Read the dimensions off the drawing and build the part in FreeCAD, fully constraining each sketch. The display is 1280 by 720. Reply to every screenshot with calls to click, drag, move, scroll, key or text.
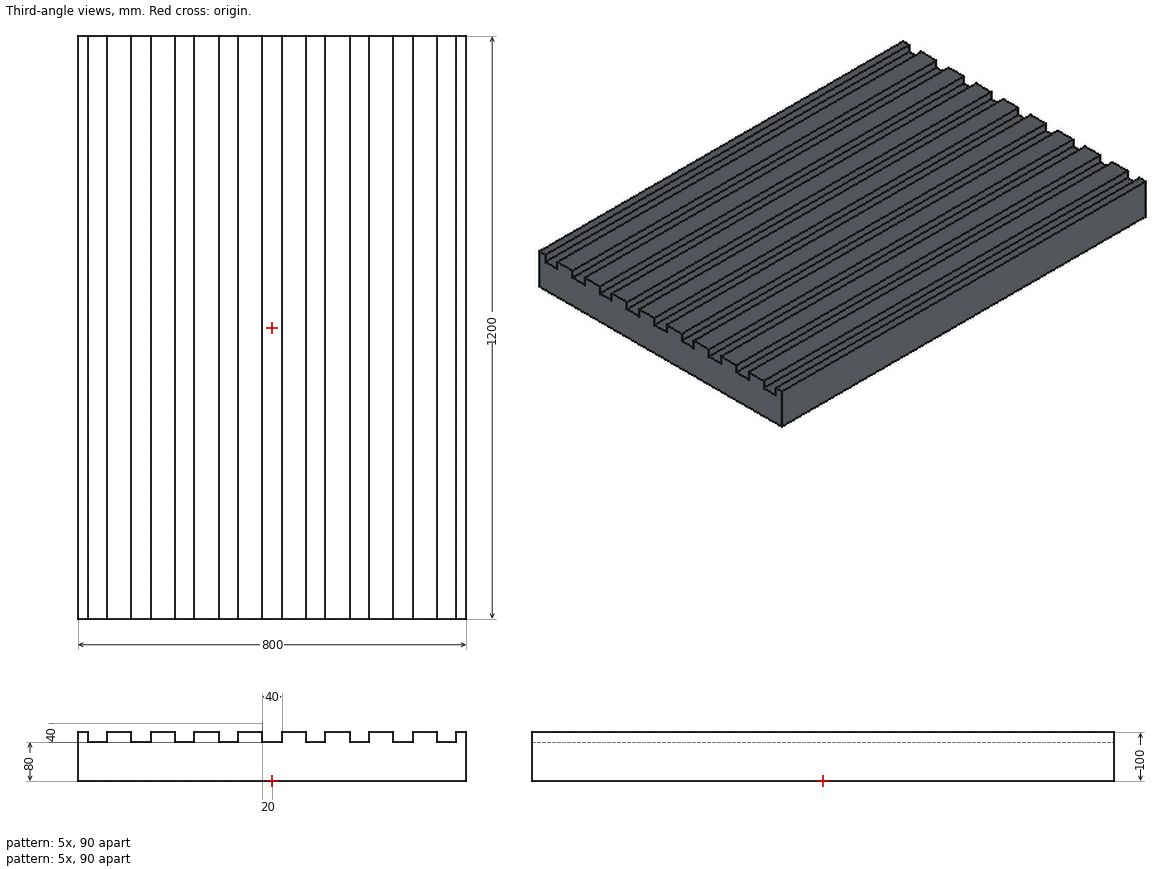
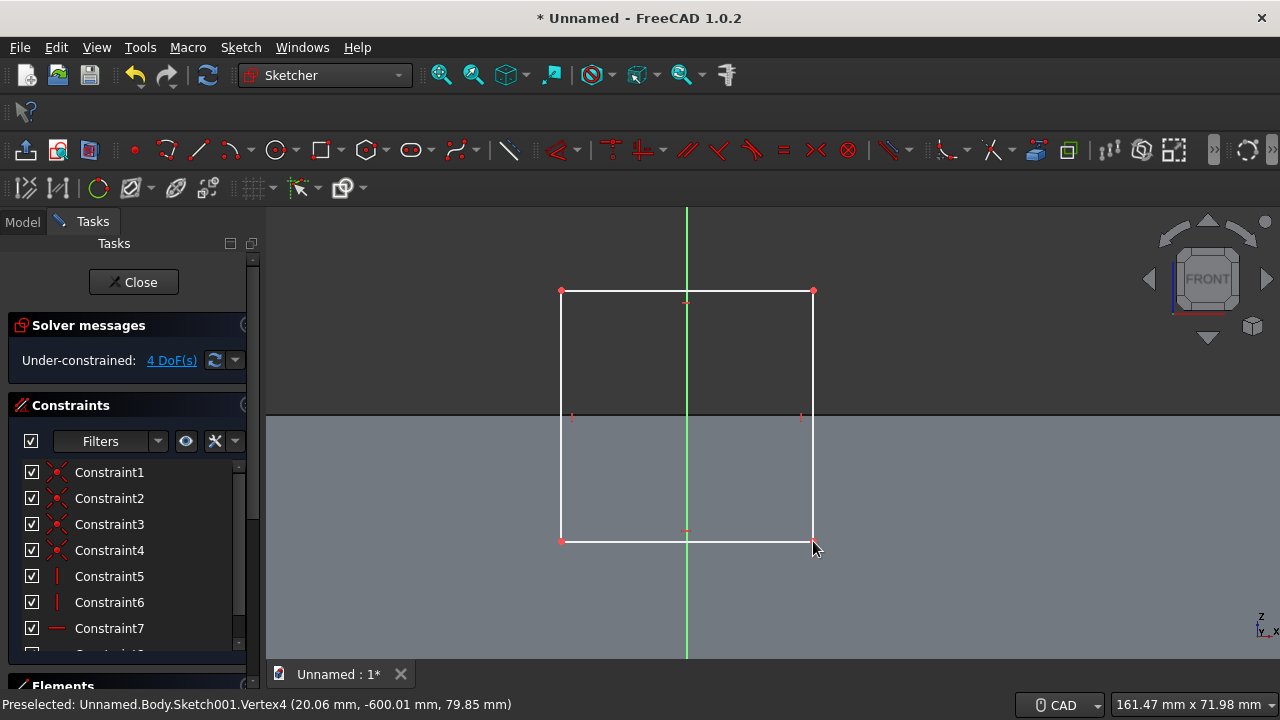
key(d)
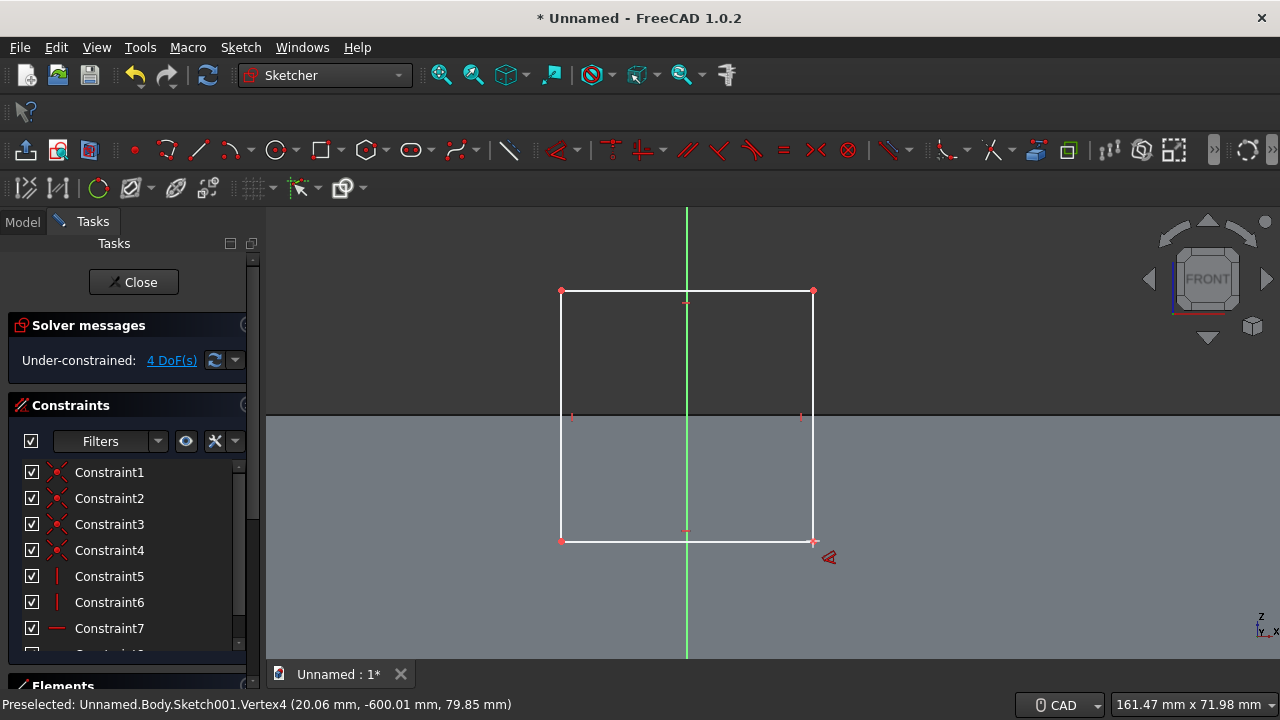
click(561, 366)
click(527, 416)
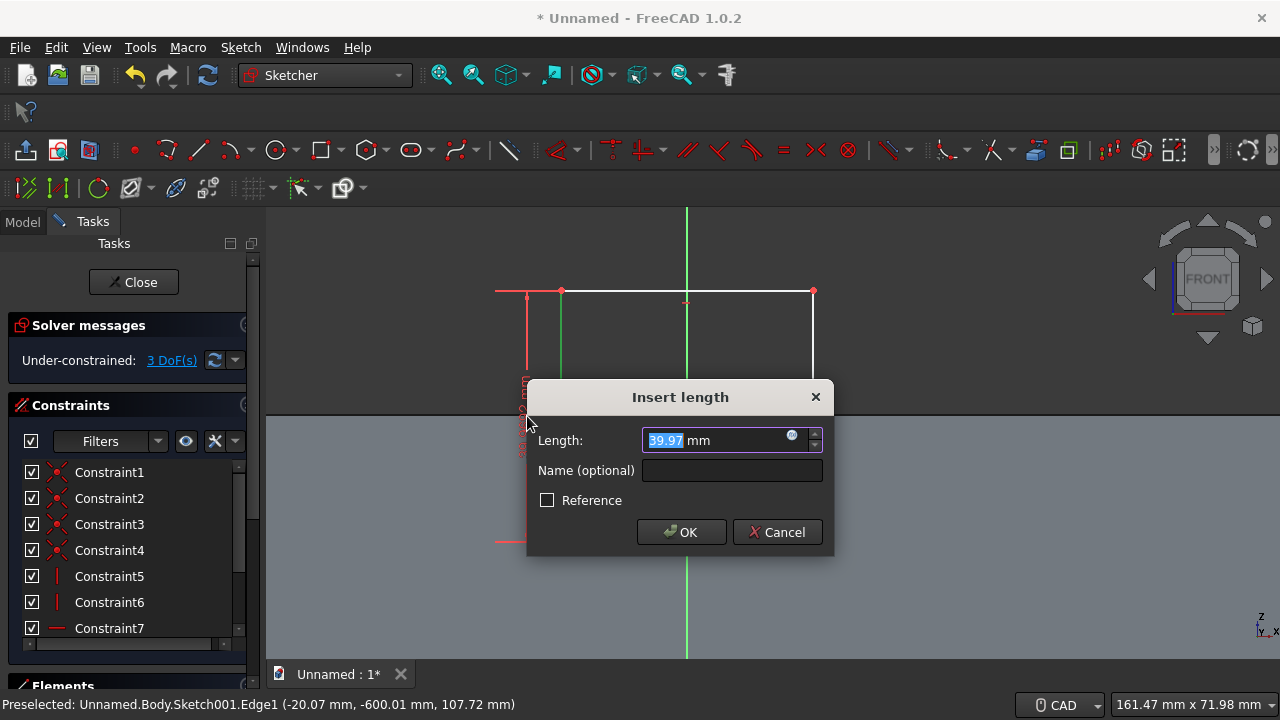
text(40)
key(Return)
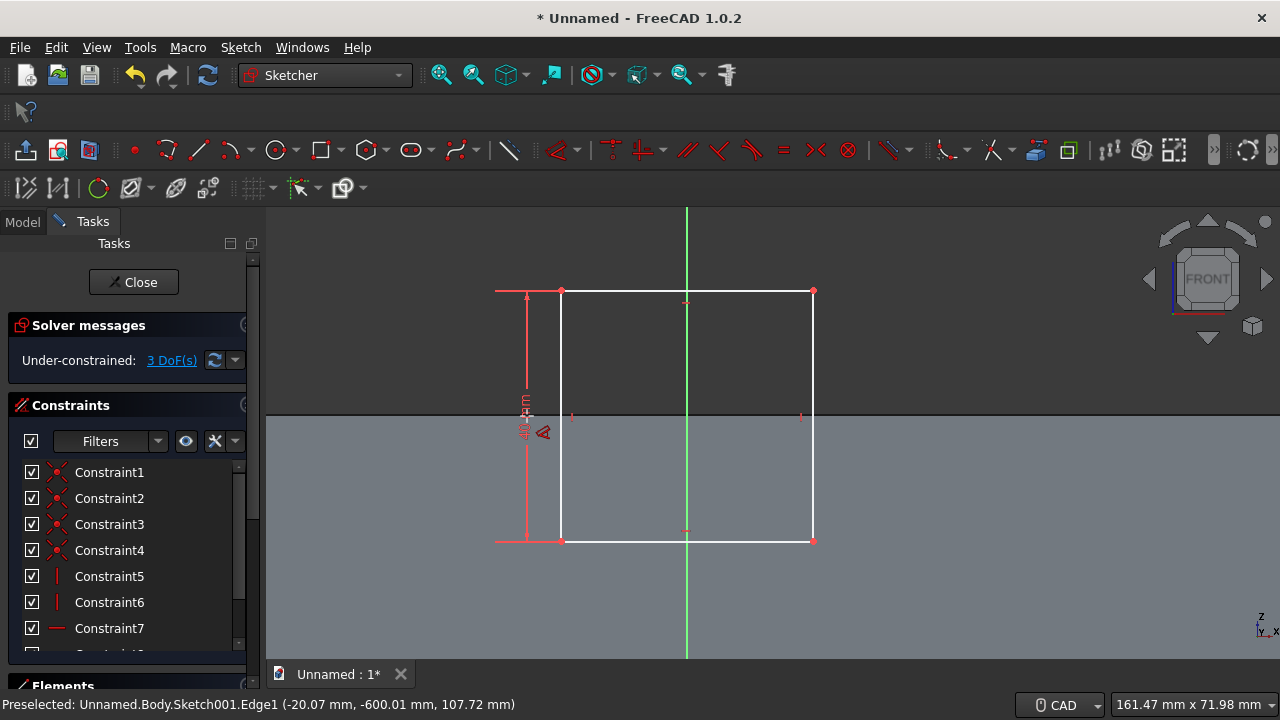
click(637, 542)
click(629, 576)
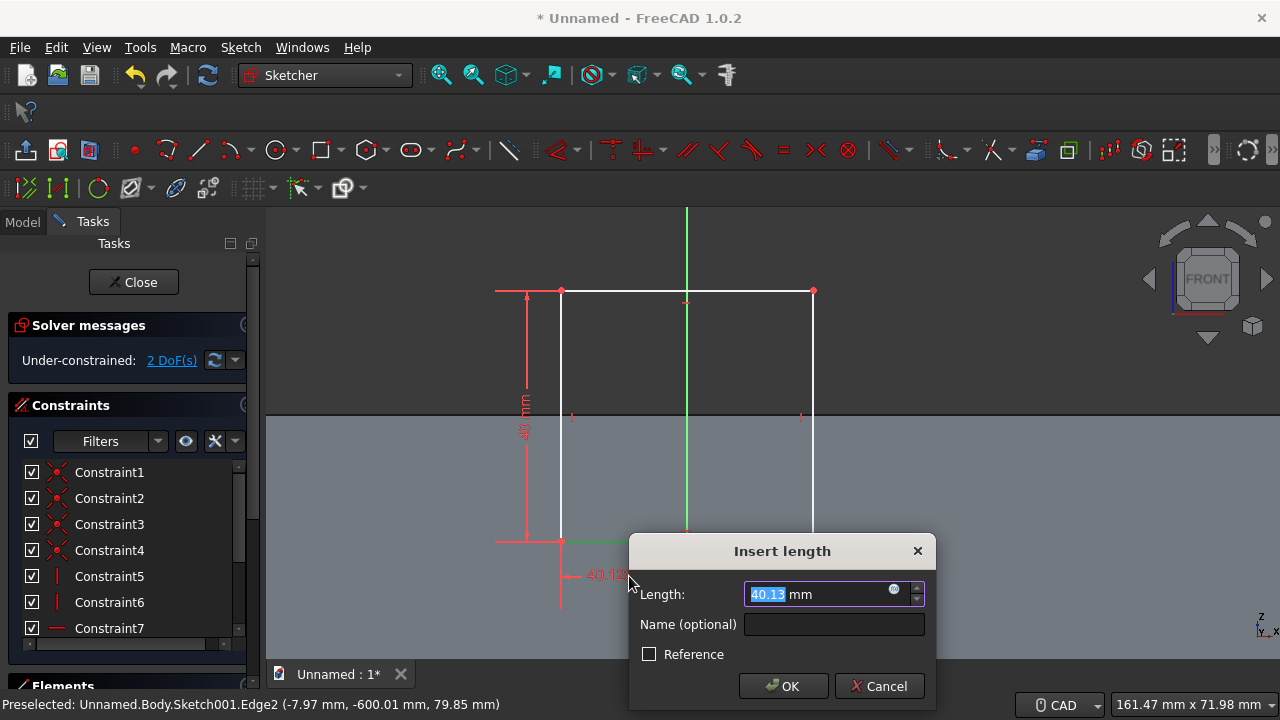
text(40)
key(Return)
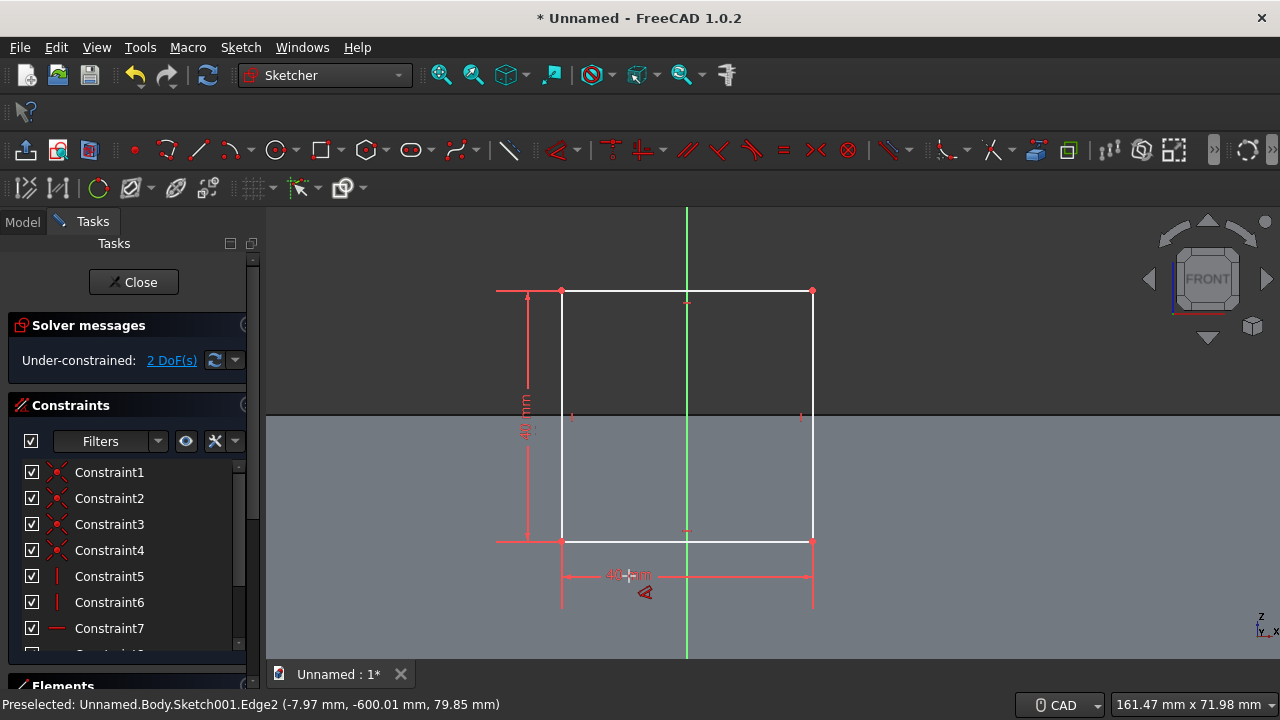
click(562, 291)
click(624, 257)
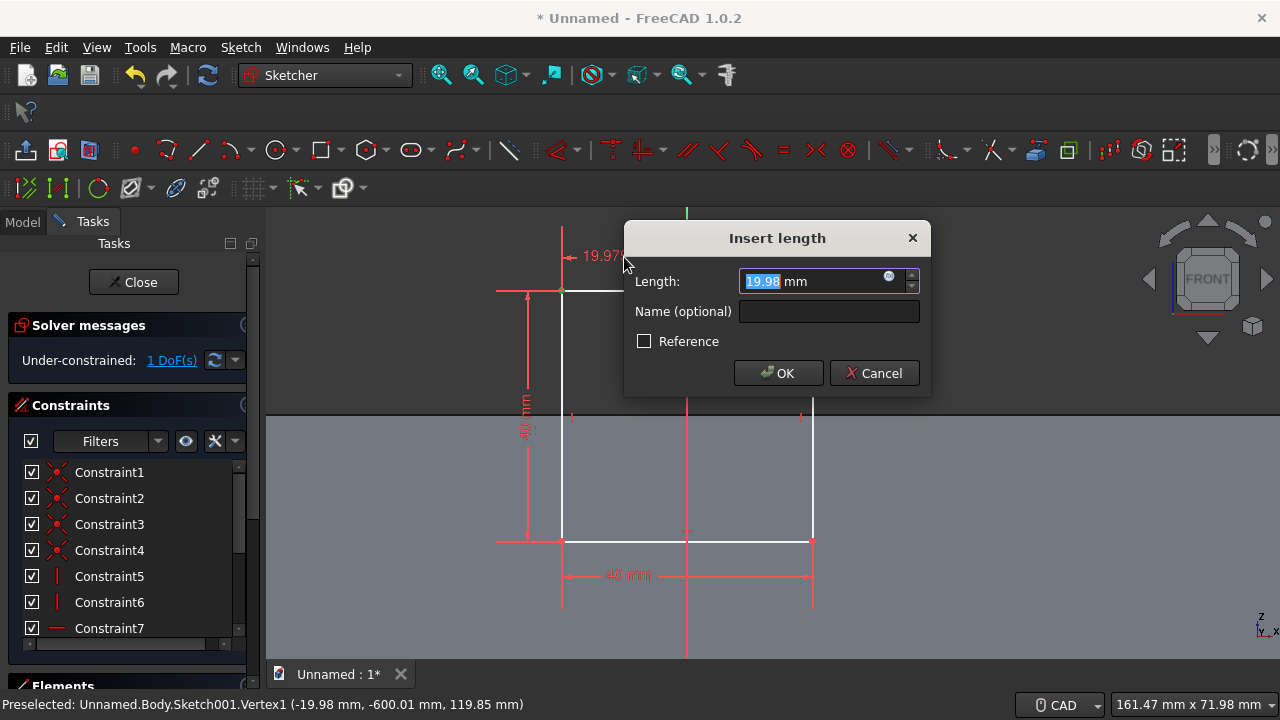
text(20)
key(Return)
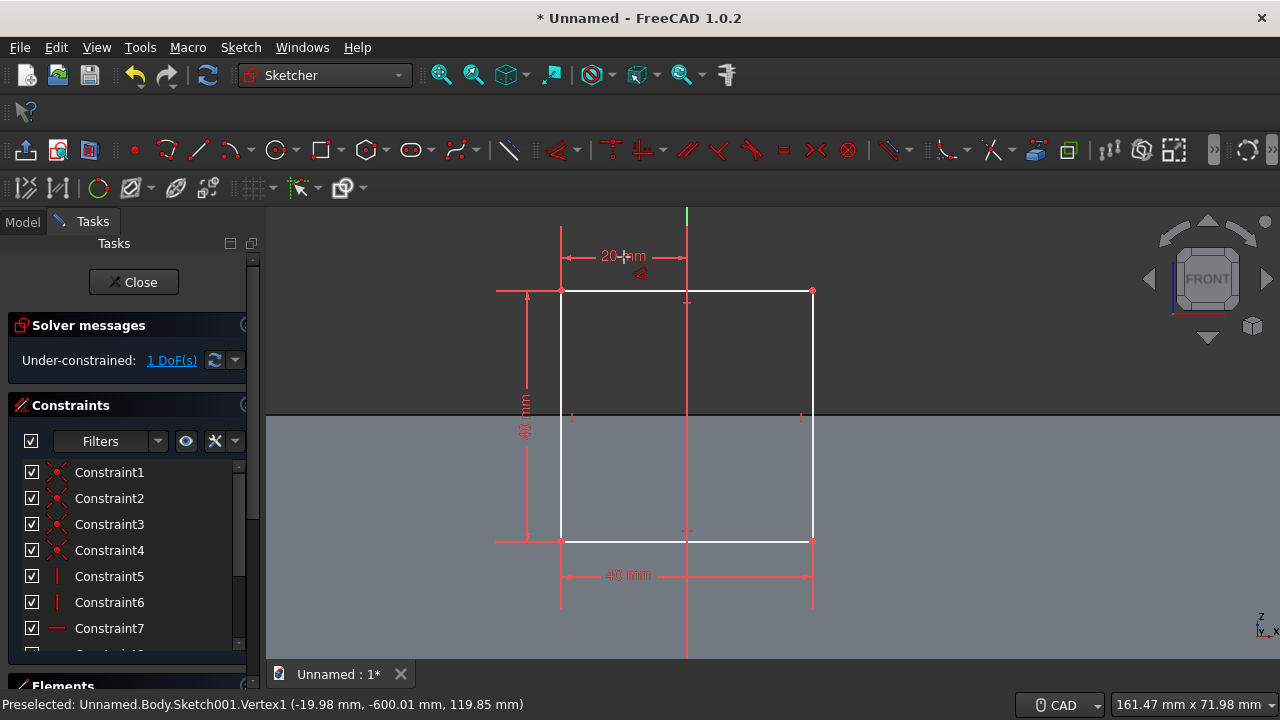
click(561, 542)
click(527, 586)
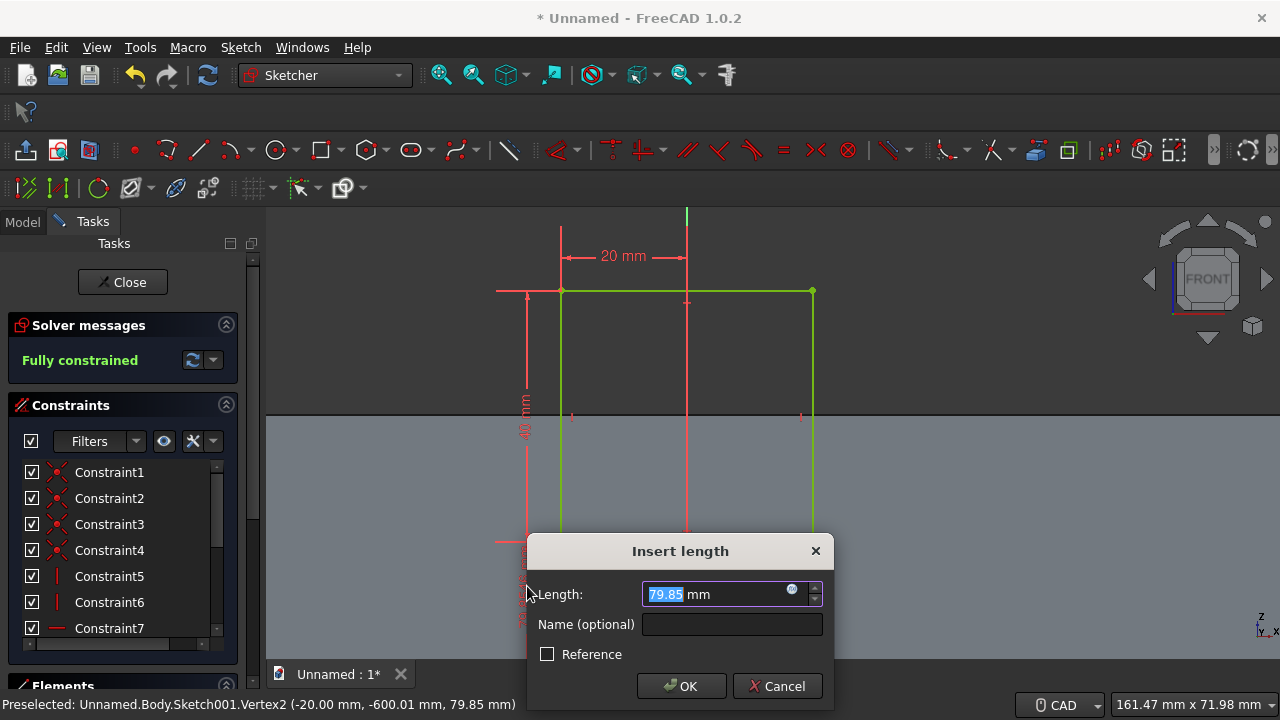
text(80)
key(Return)
key(Escape)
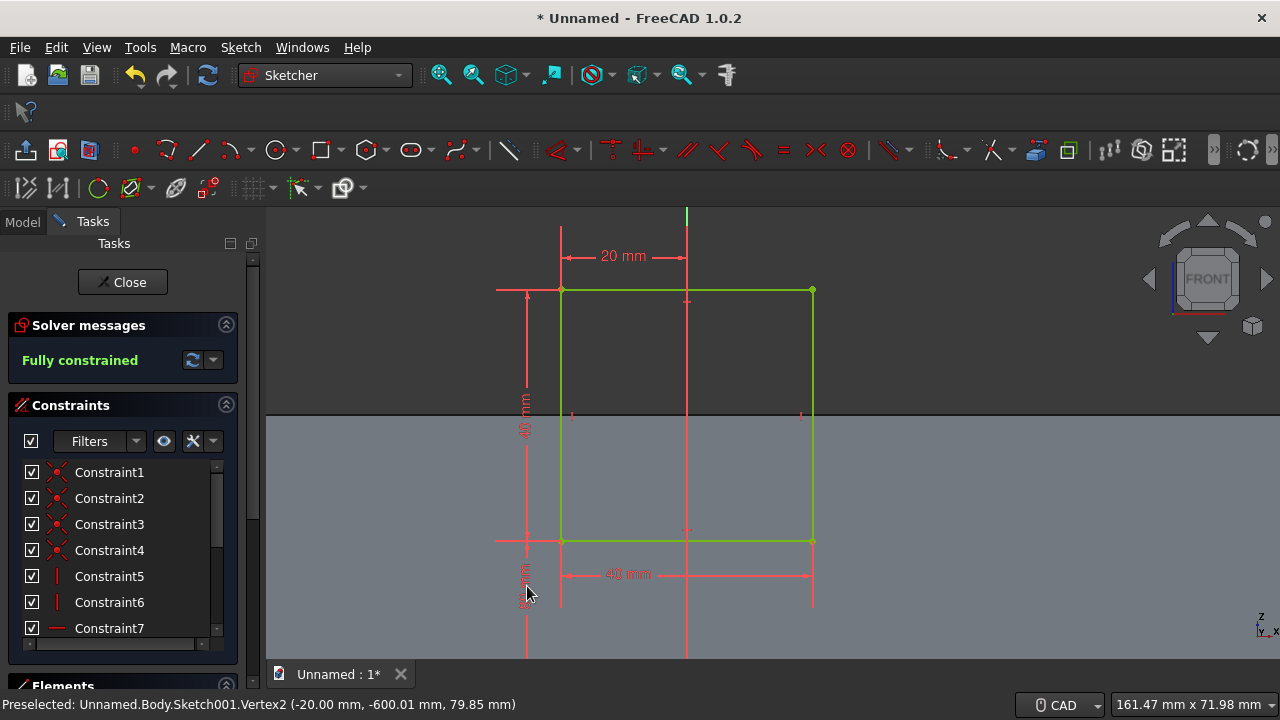
click(123, 282)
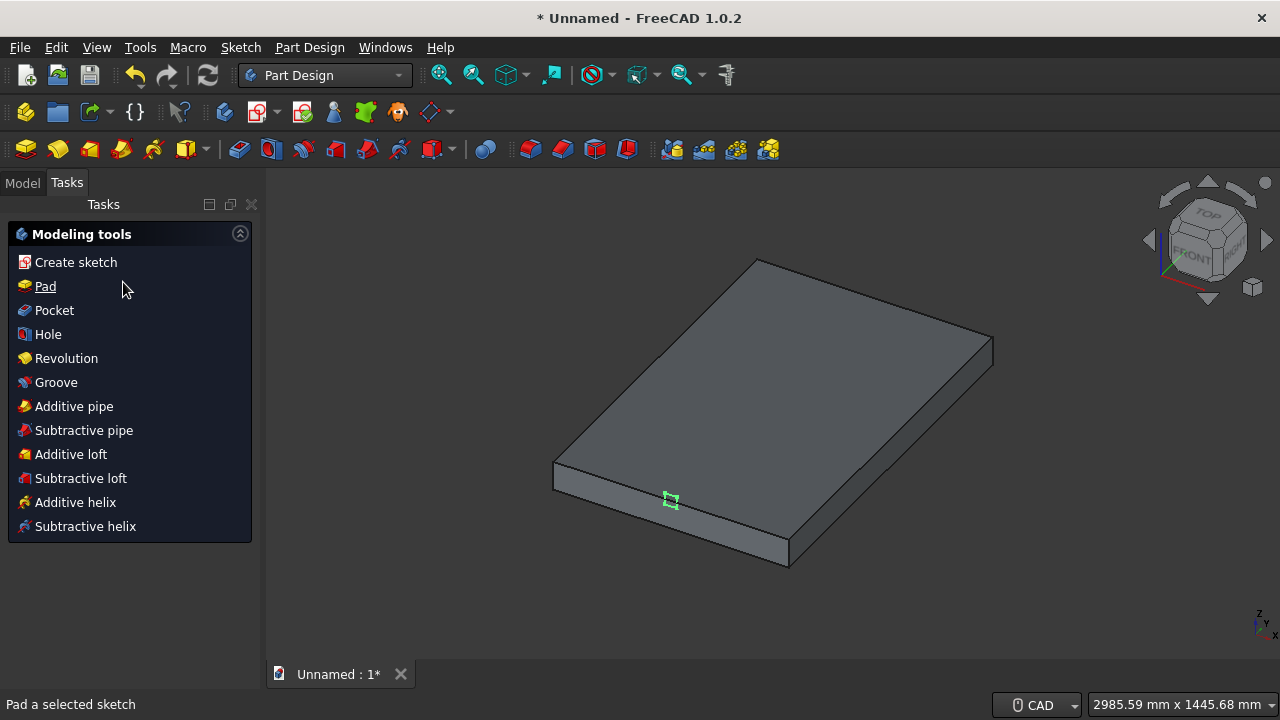
click(240, 150)